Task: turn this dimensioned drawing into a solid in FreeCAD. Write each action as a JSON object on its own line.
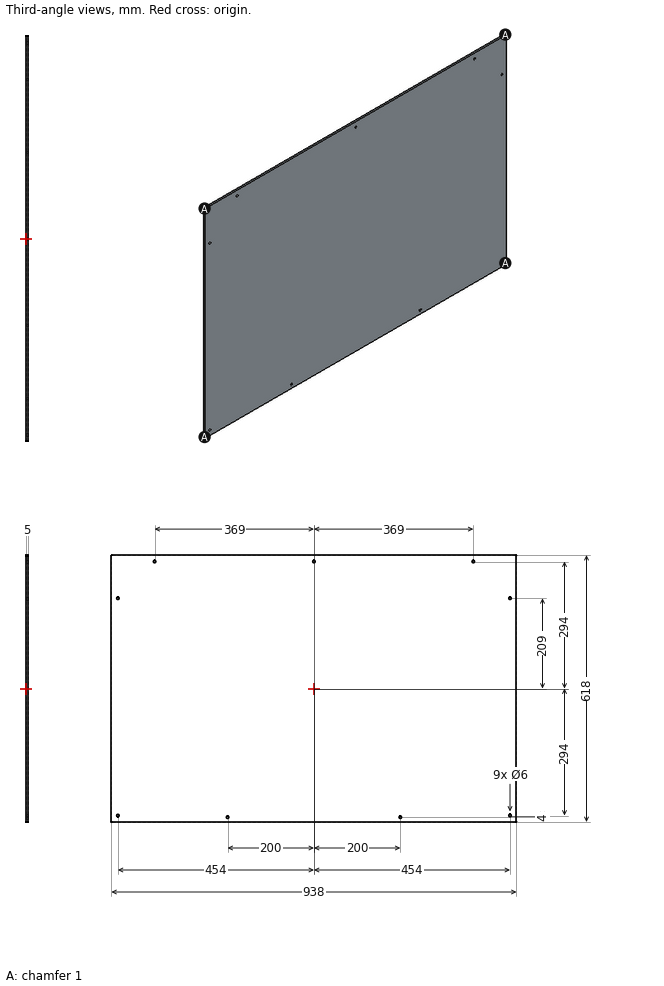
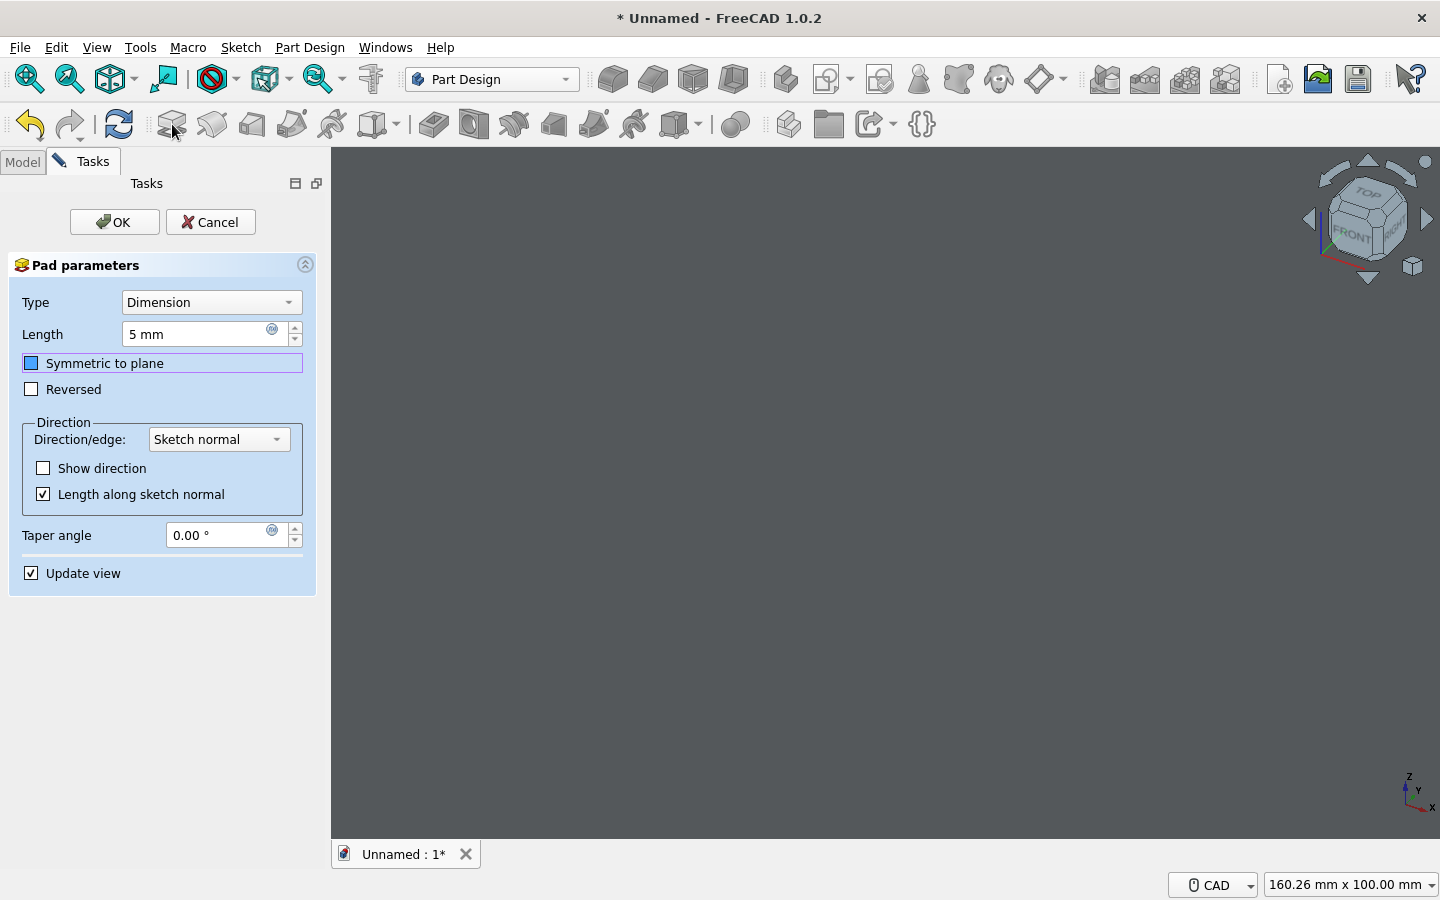
{"action": "left_click", "coordinate": [115, 222]}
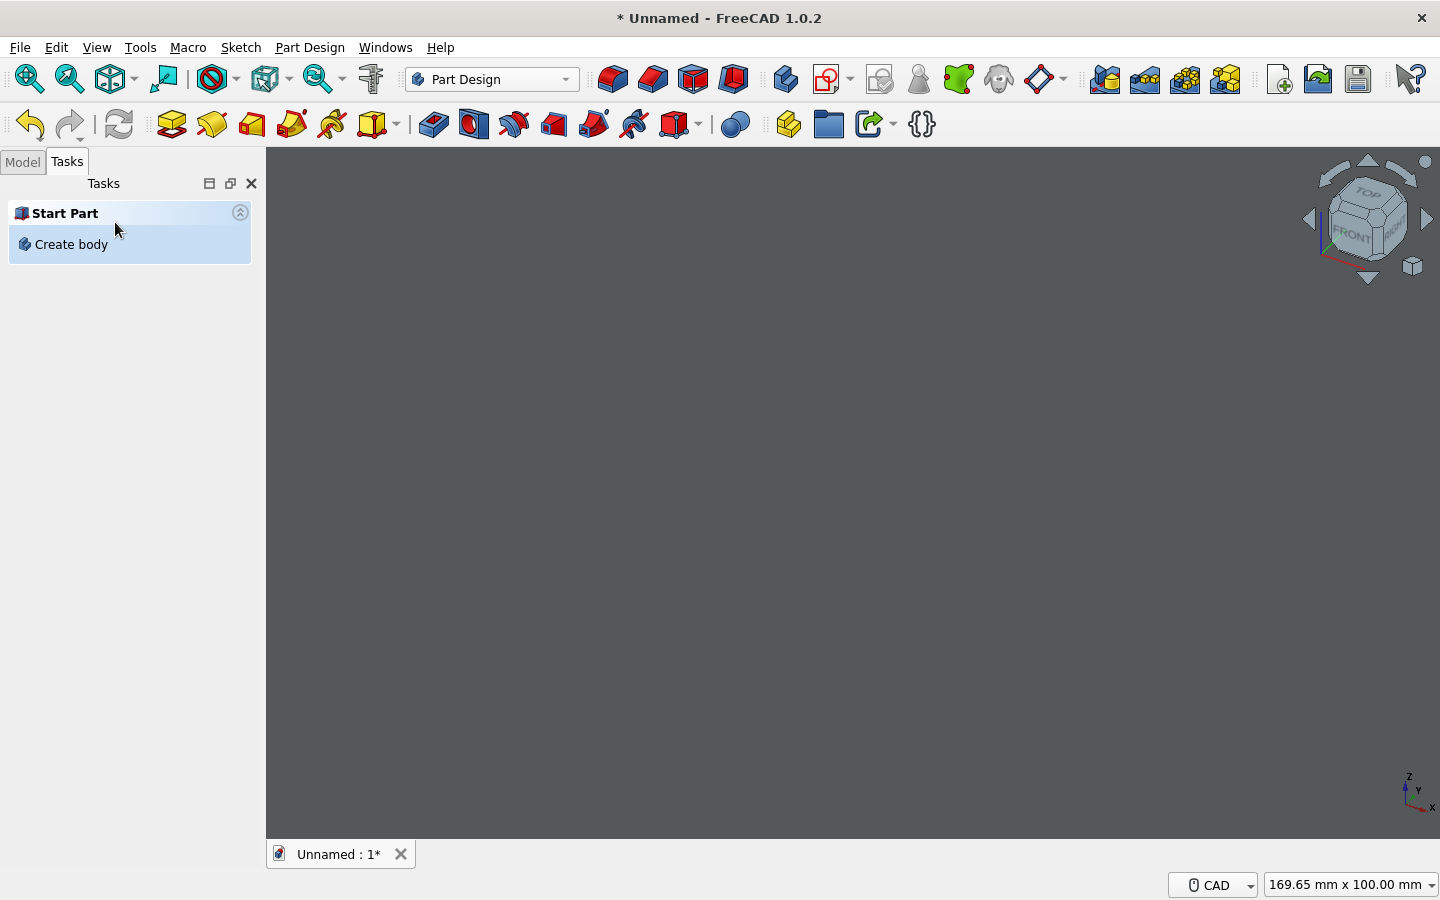
{"action": "left_click", "coordinate": [30, 80]}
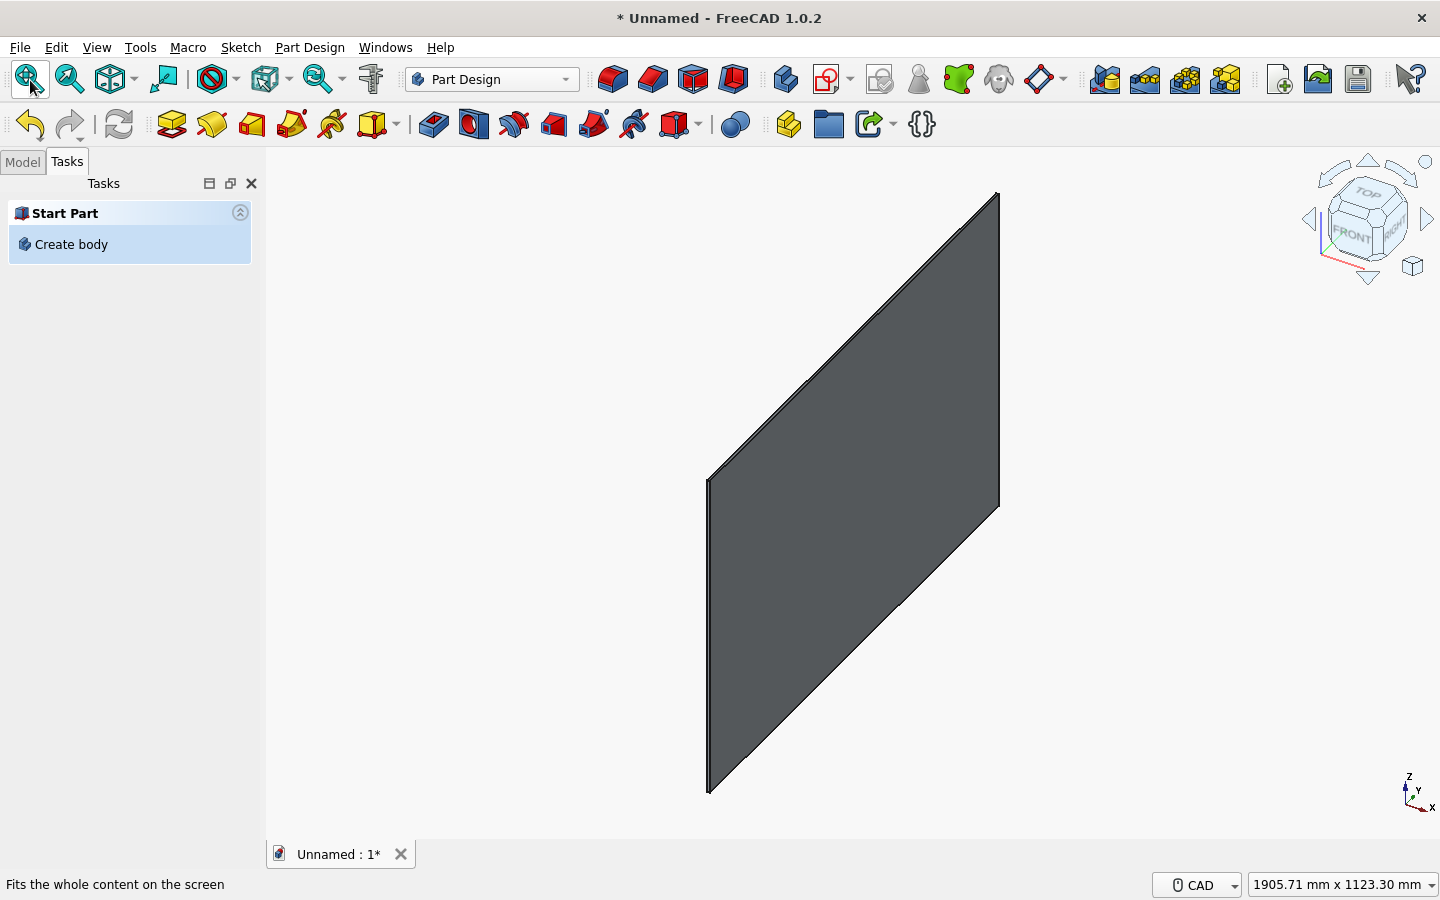
{"action": "scroll", "coordinate": [997, 193], "scroll_direction": "up", "scroll_amount": 13}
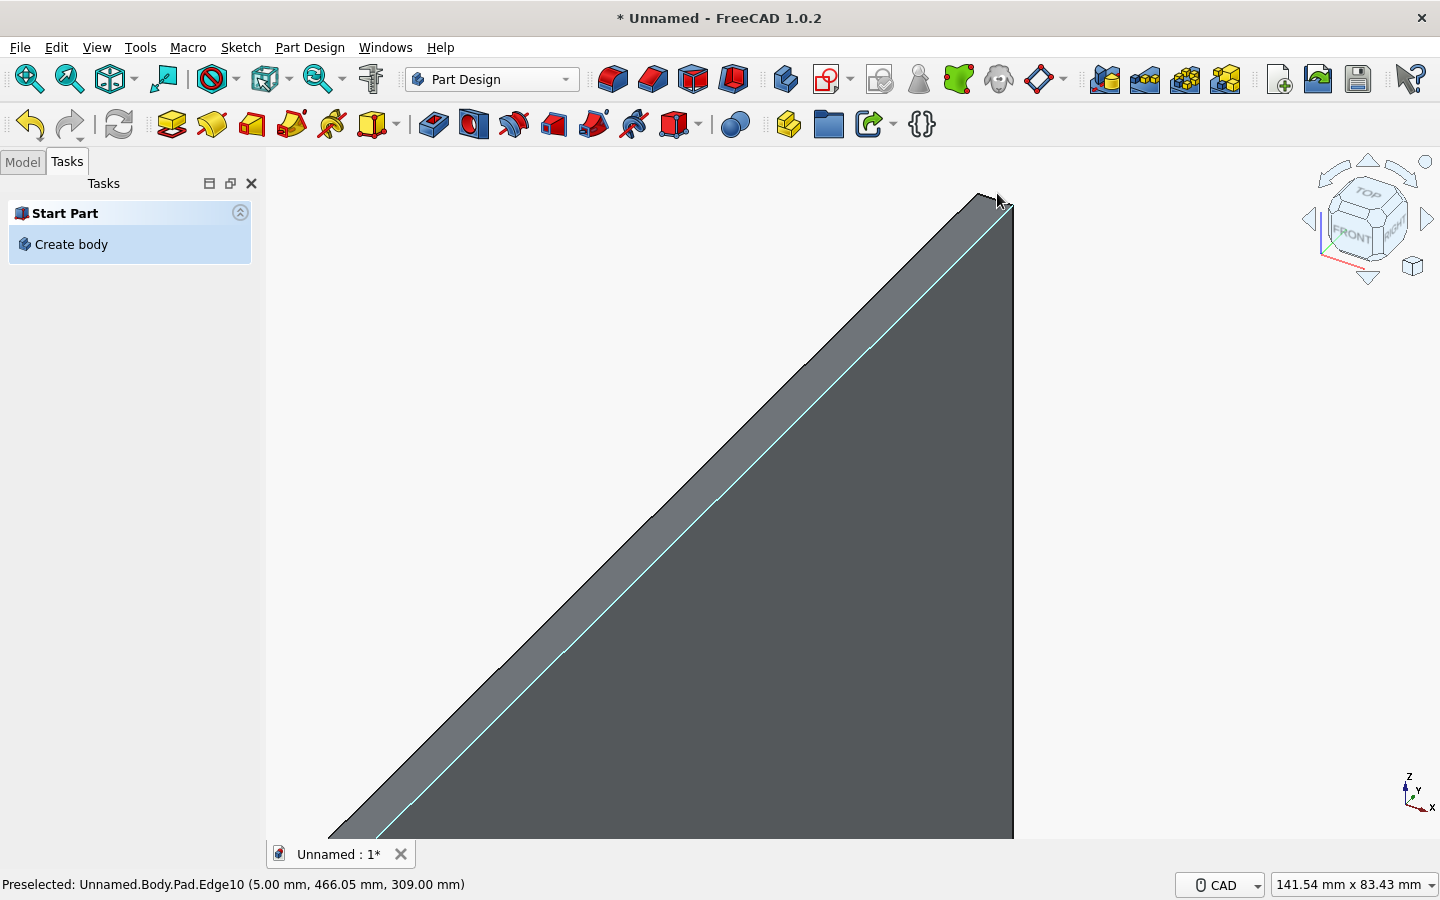
{"action": "left_click", "coordinate": [30, 80]}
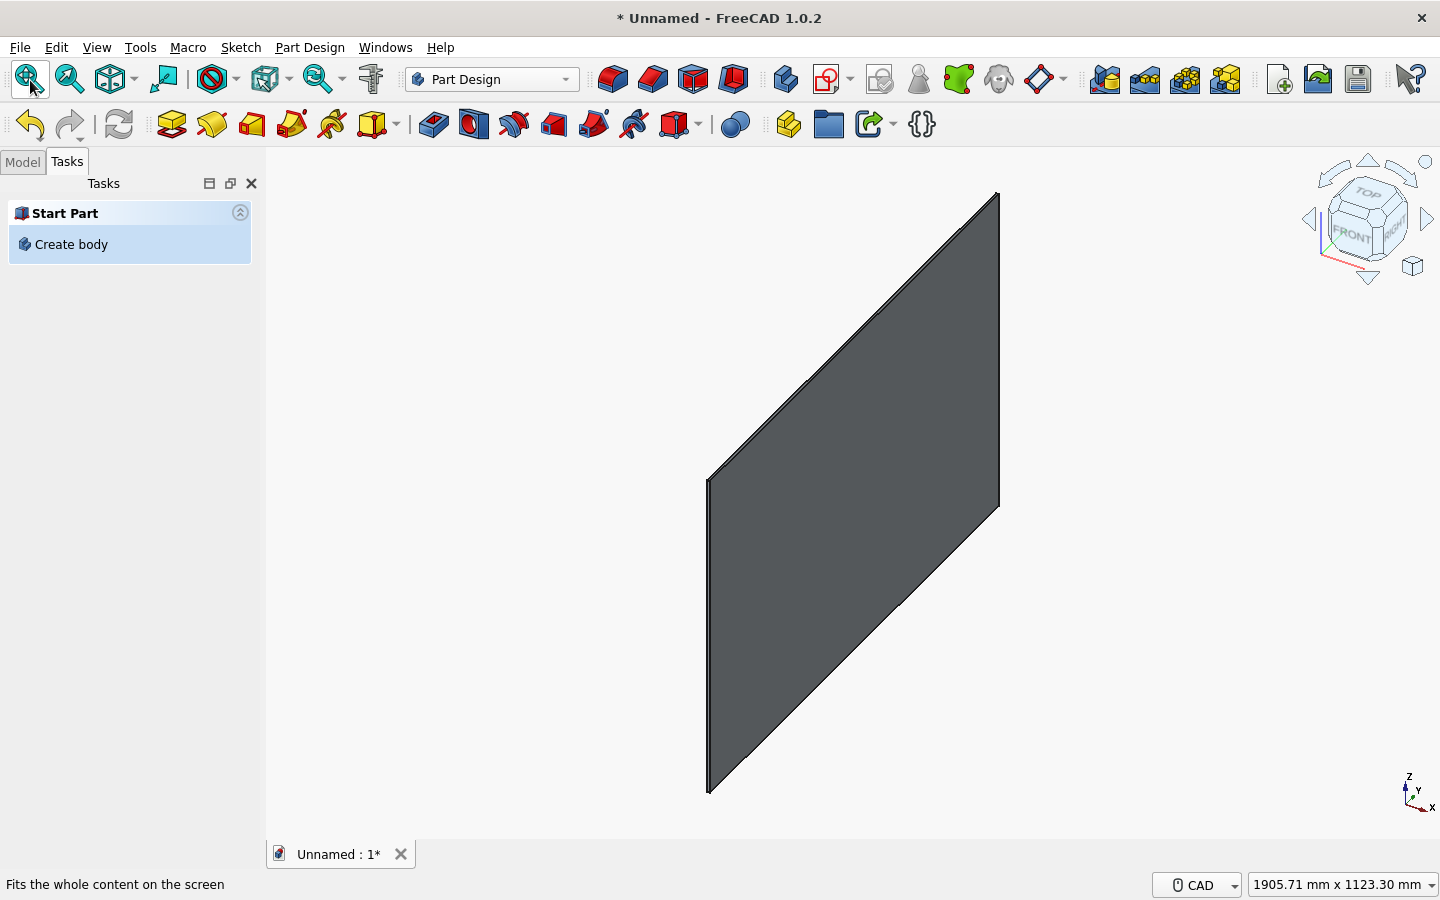
{"action": "key", "text": "0"}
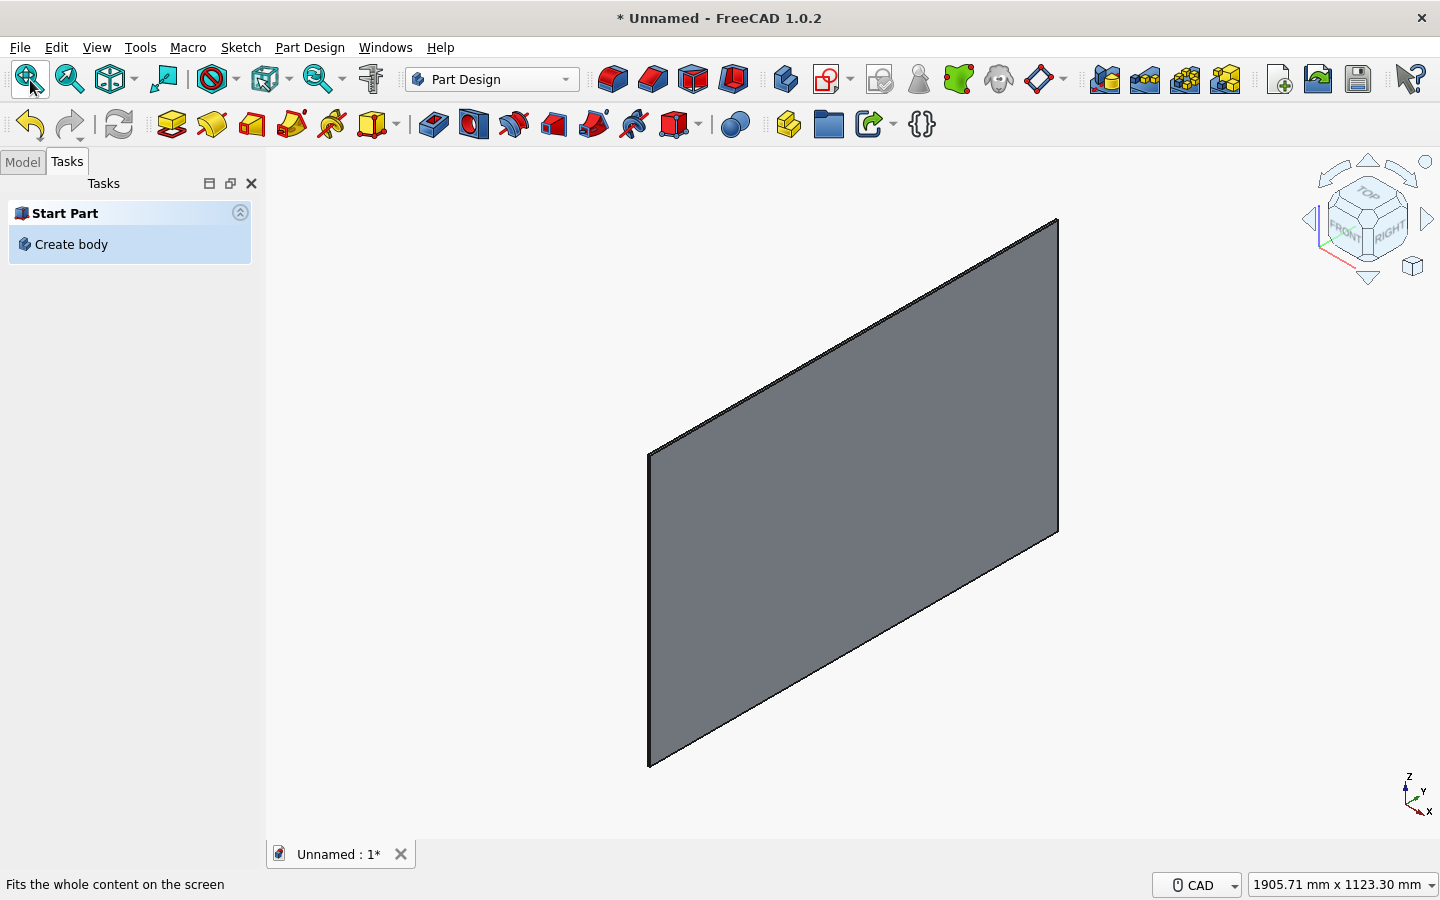
{"action": "scroll", "coordinate": [1057, 219], "scroll_direction": "up", "scroll_amount": 13}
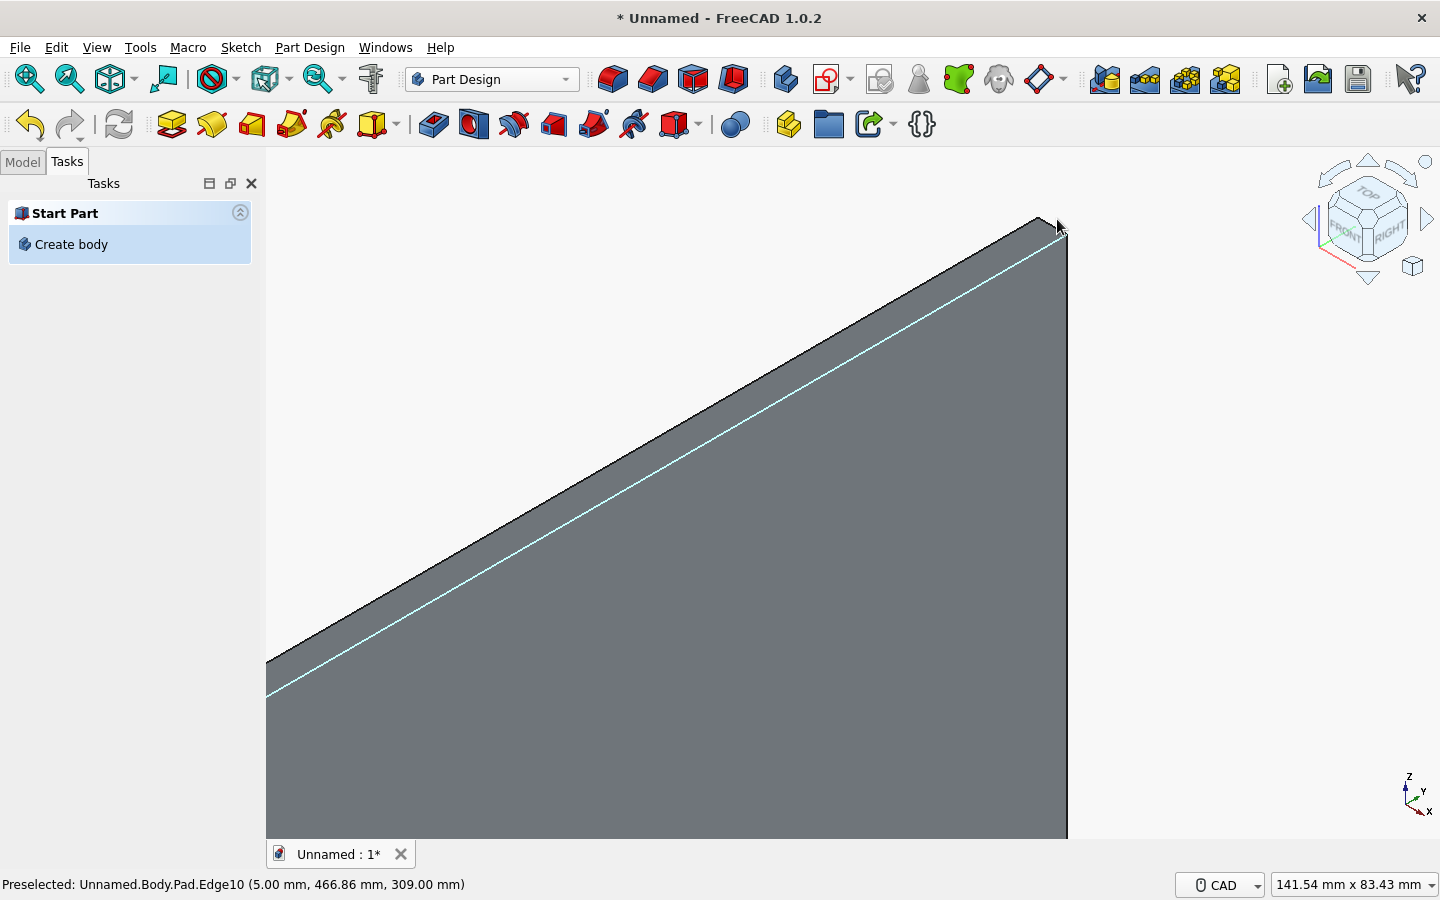
{"action": "left_click", "coordinate": [30, 80]}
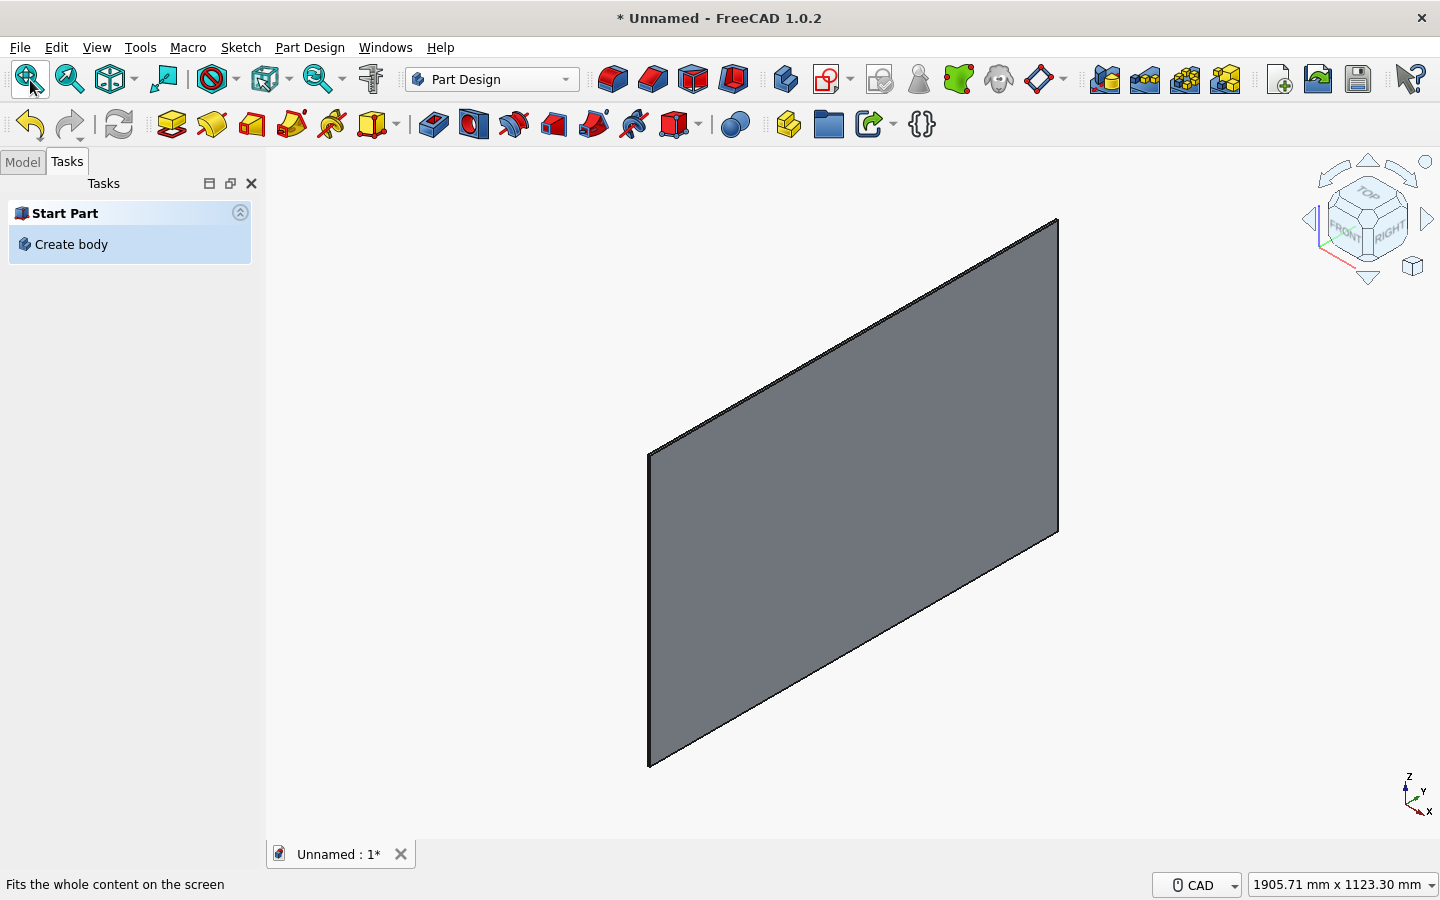
{"action": "key", "text": "2"}